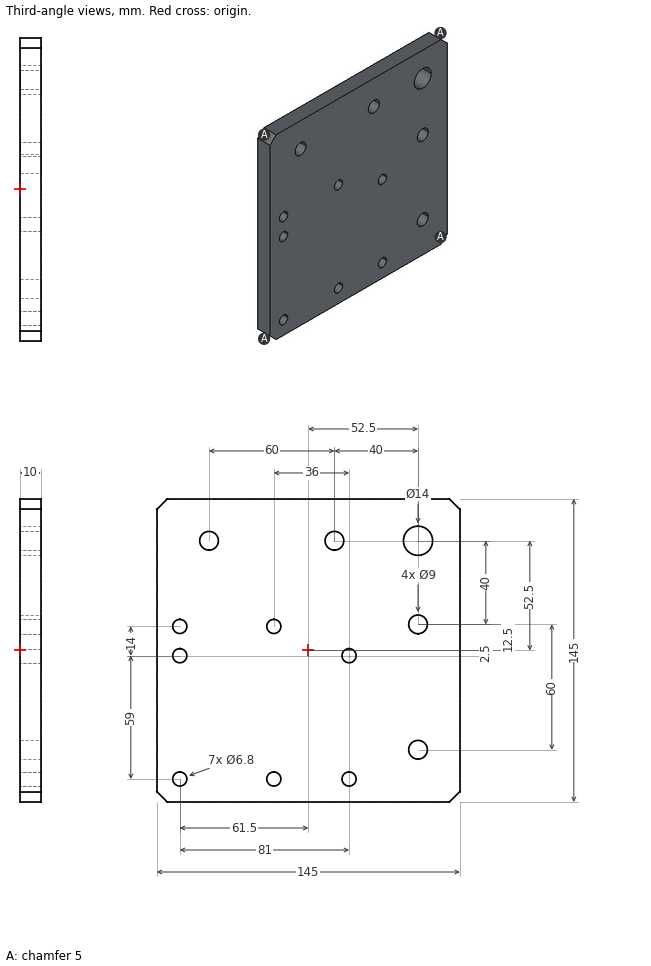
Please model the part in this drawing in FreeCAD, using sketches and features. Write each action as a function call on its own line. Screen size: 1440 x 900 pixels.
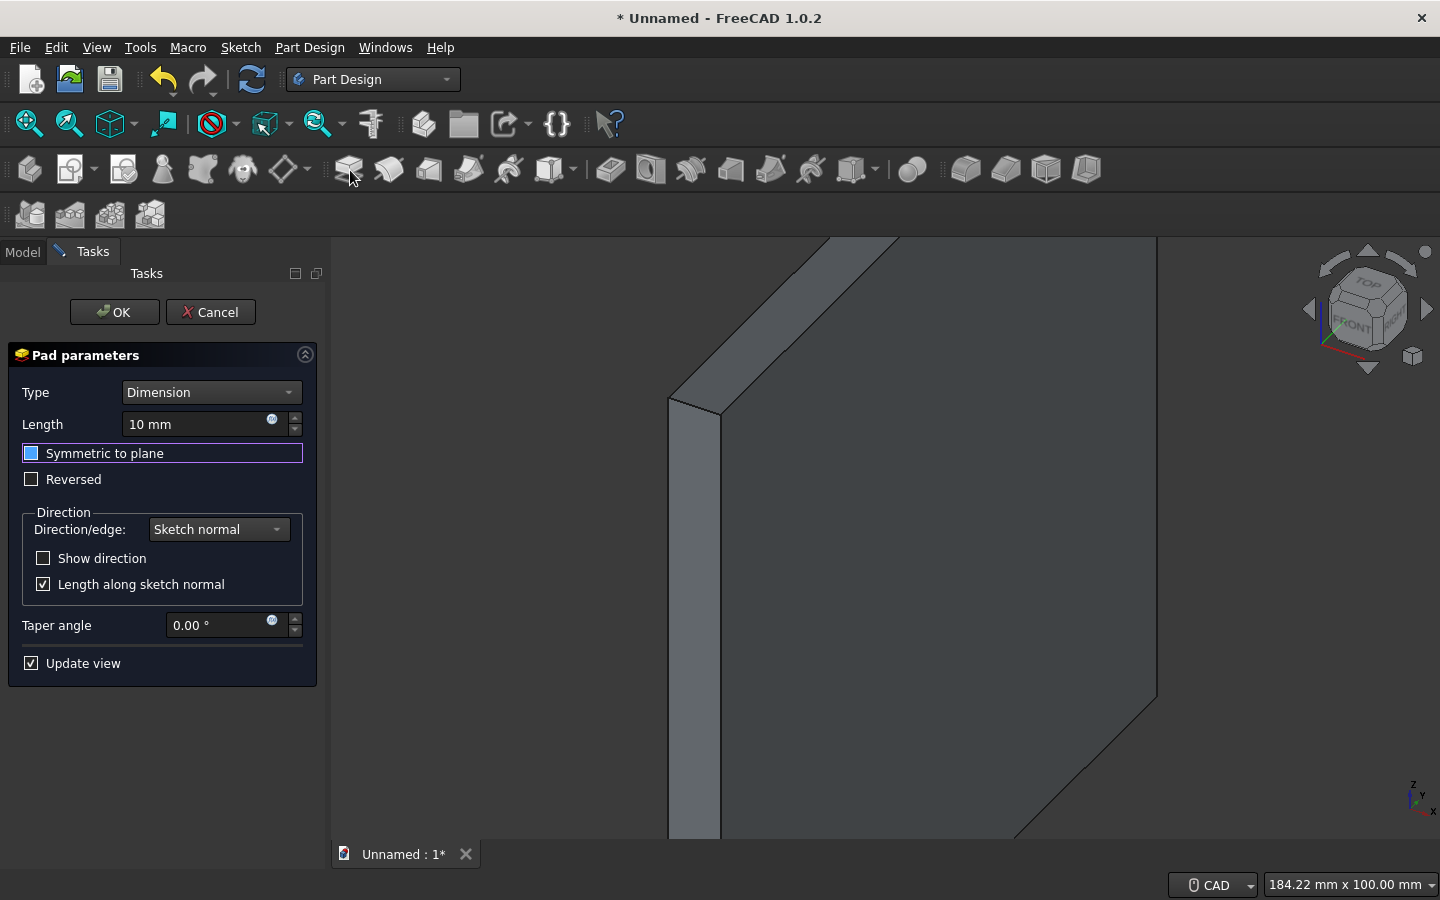
click(115, 312)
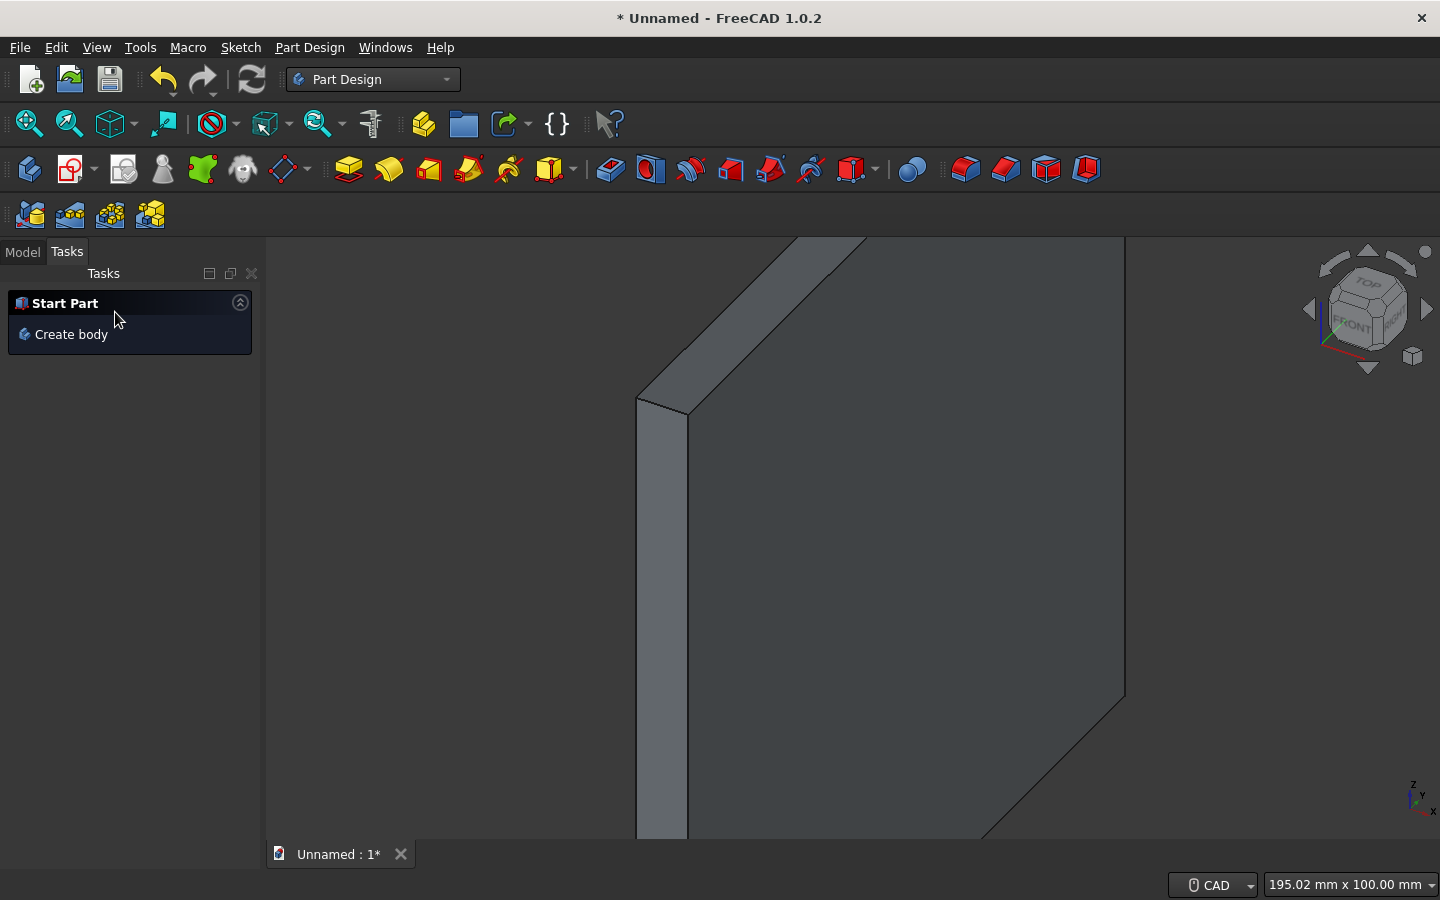
click(30, 124)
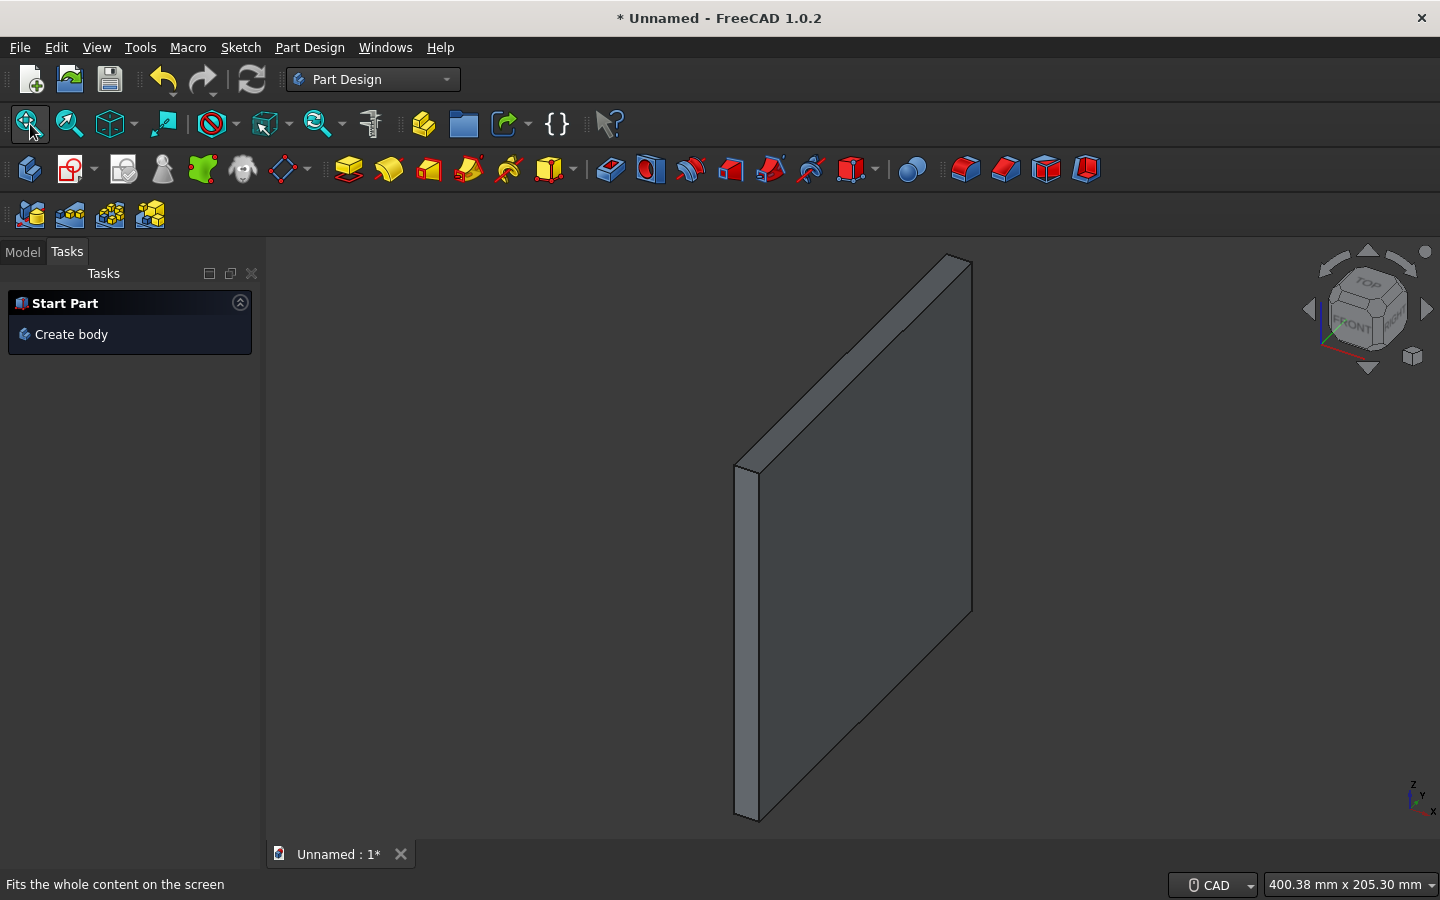
click(747, 468)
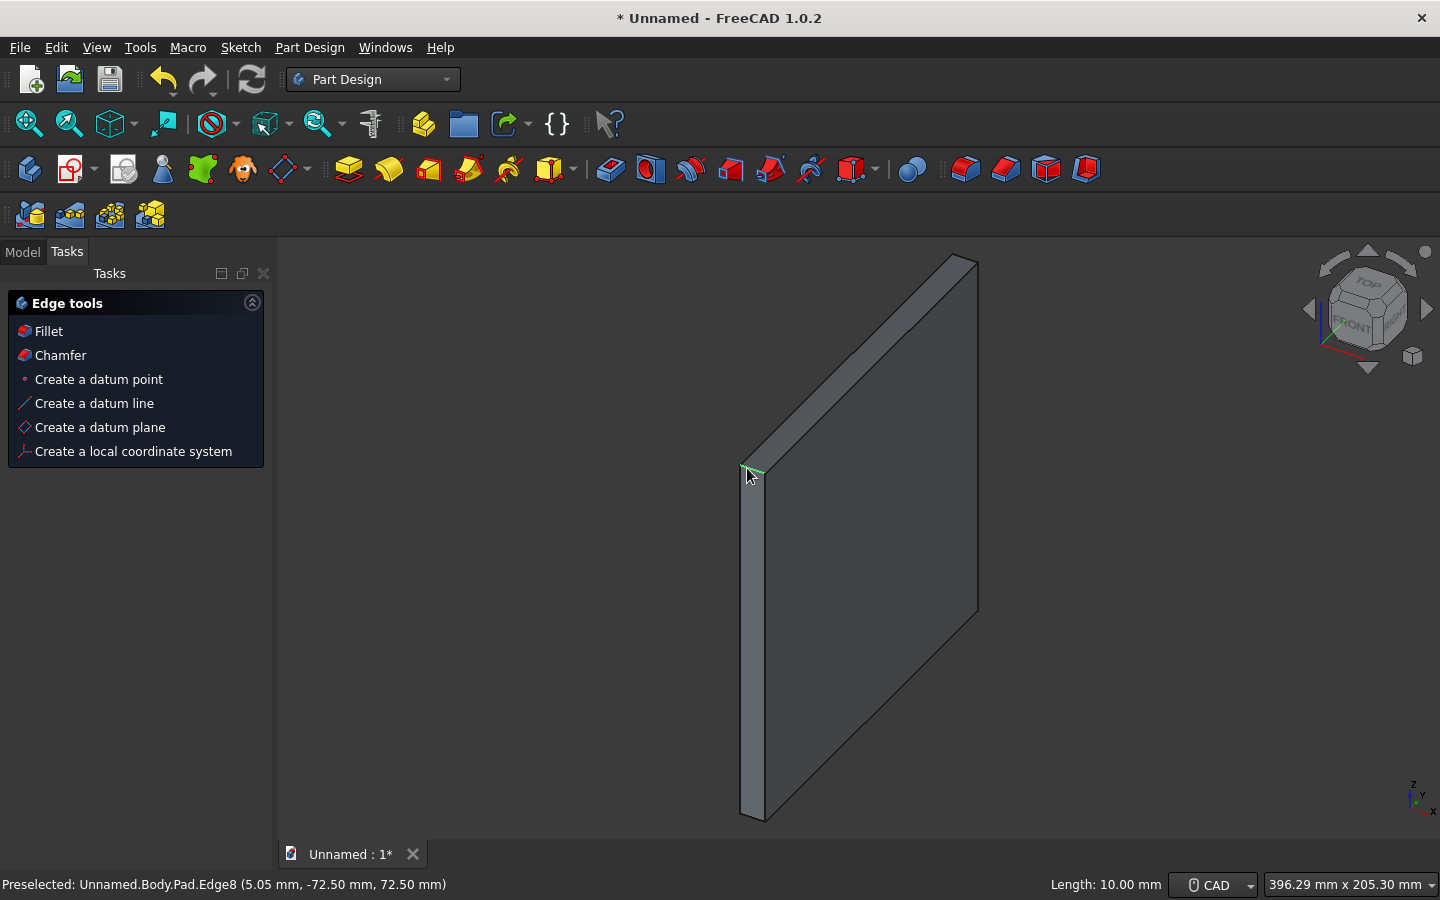
key(0)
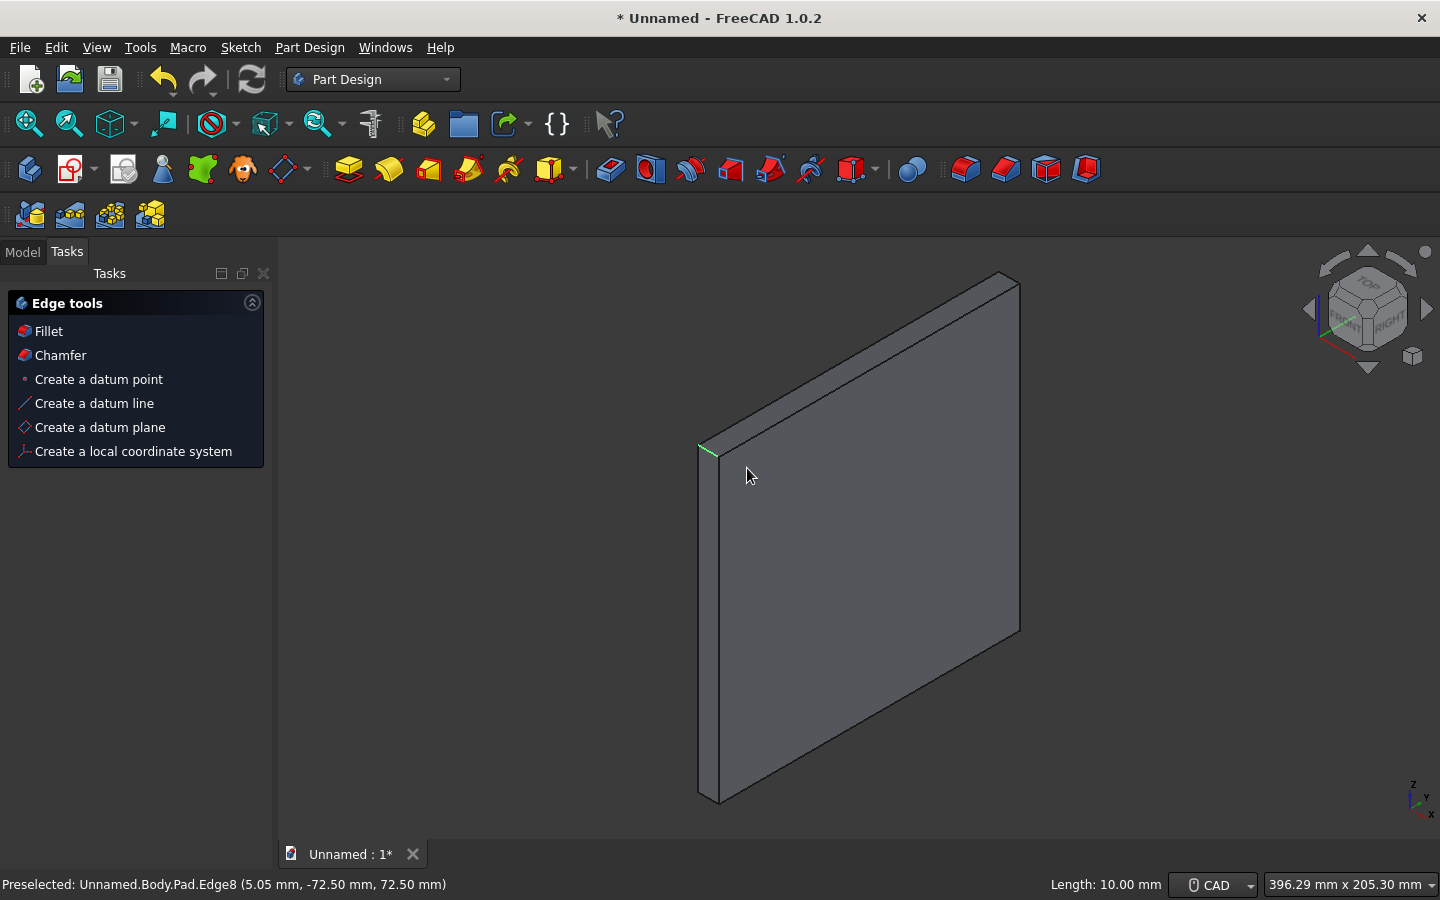
key(2)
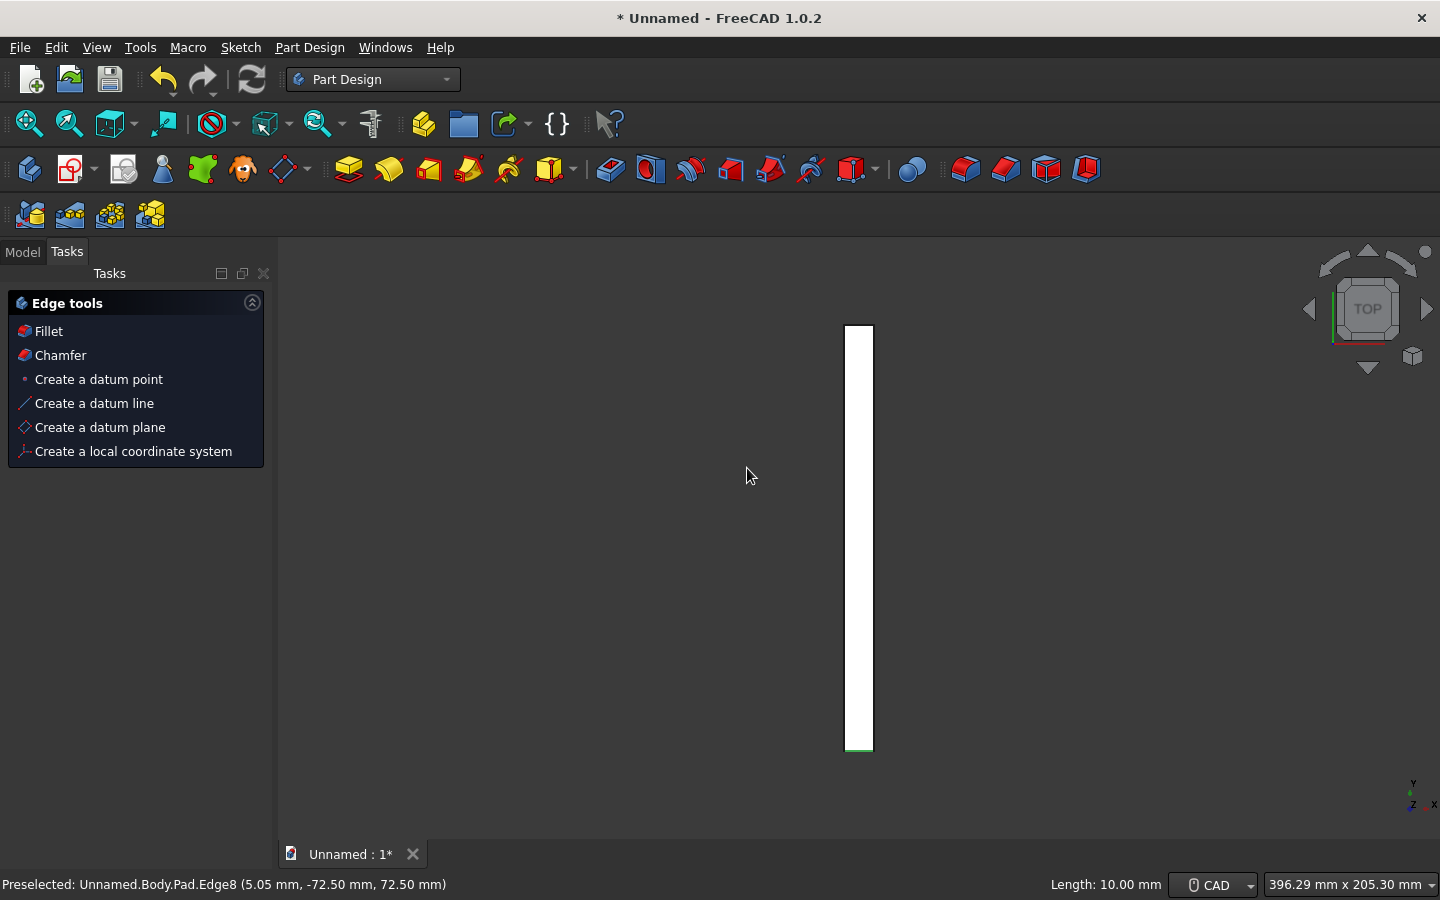
click(859, 324, ctrl)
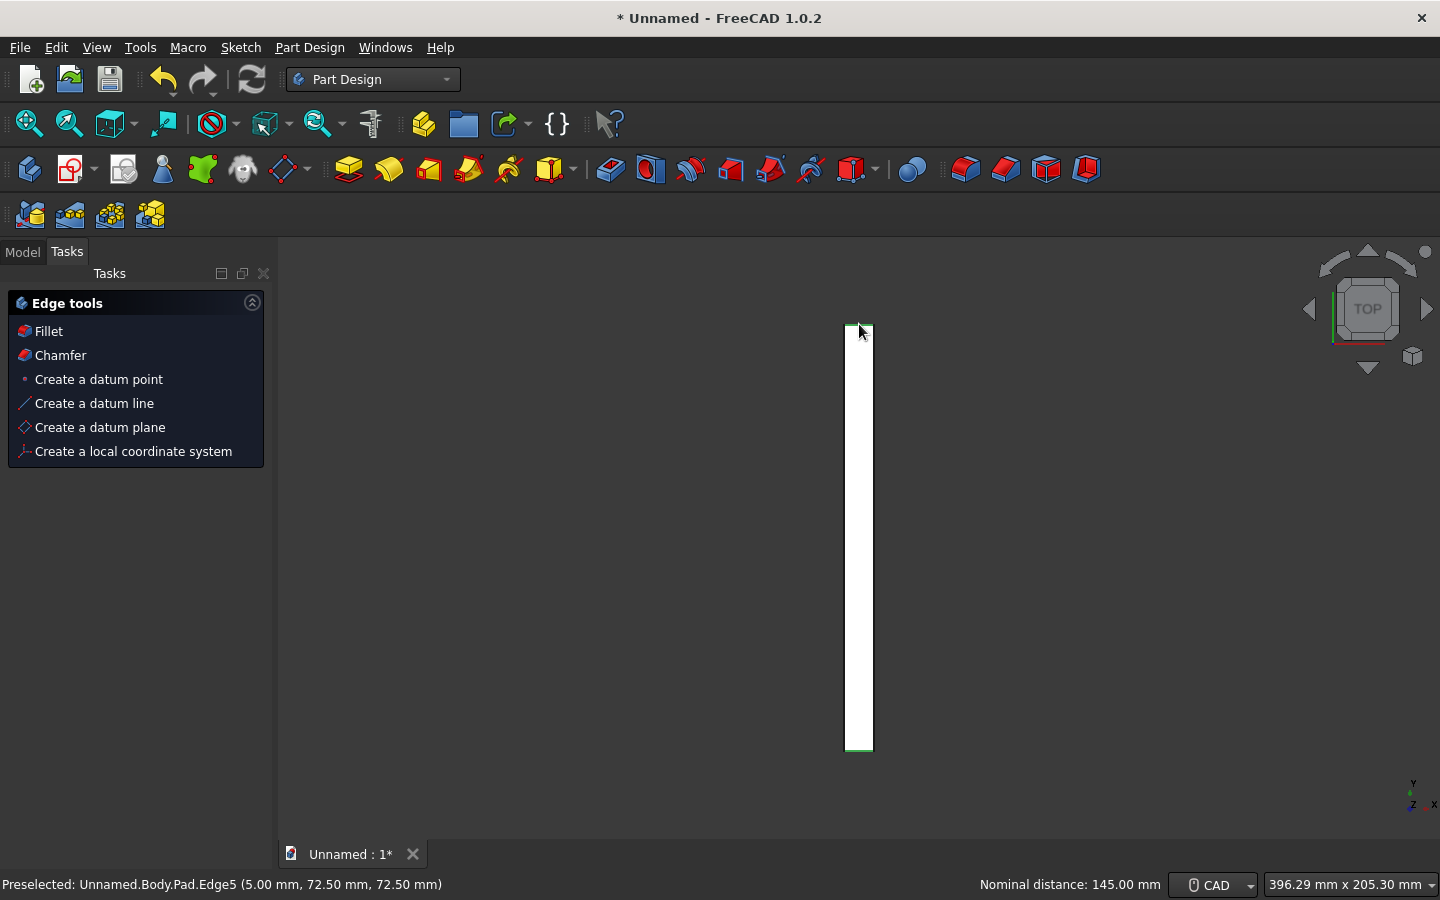
key(1)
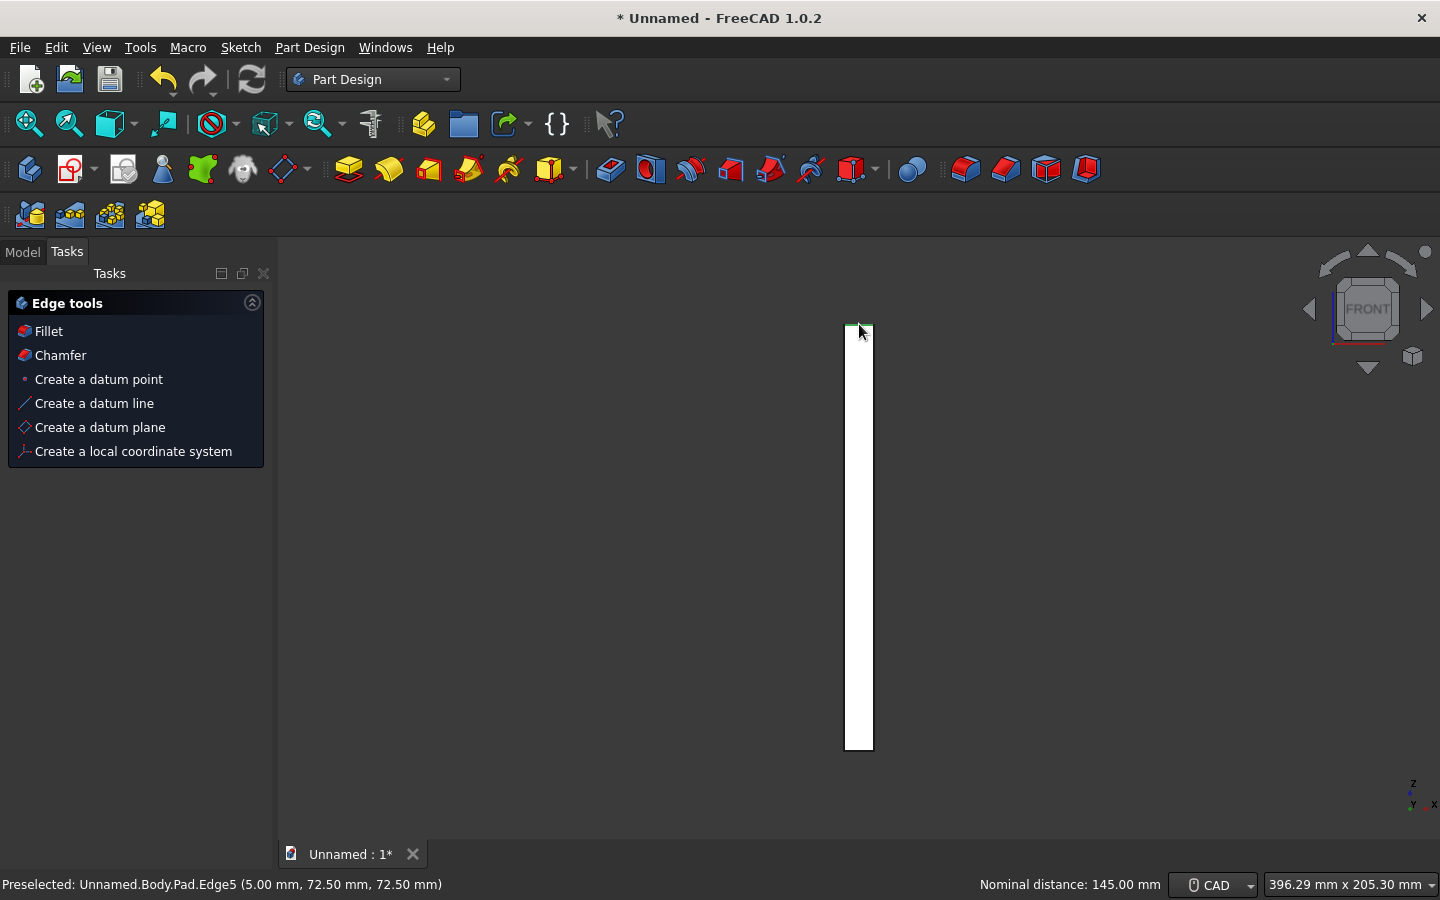
click(859, 750, ctrl)